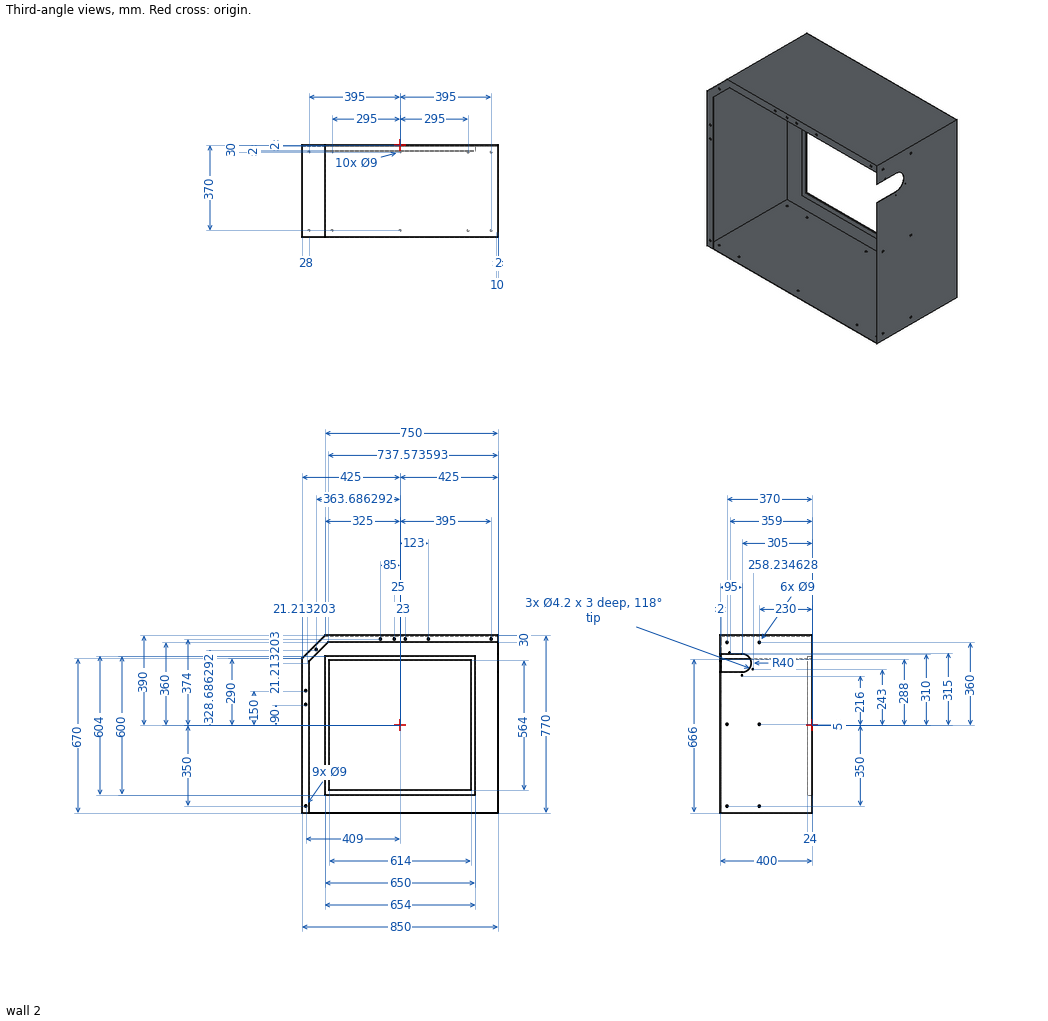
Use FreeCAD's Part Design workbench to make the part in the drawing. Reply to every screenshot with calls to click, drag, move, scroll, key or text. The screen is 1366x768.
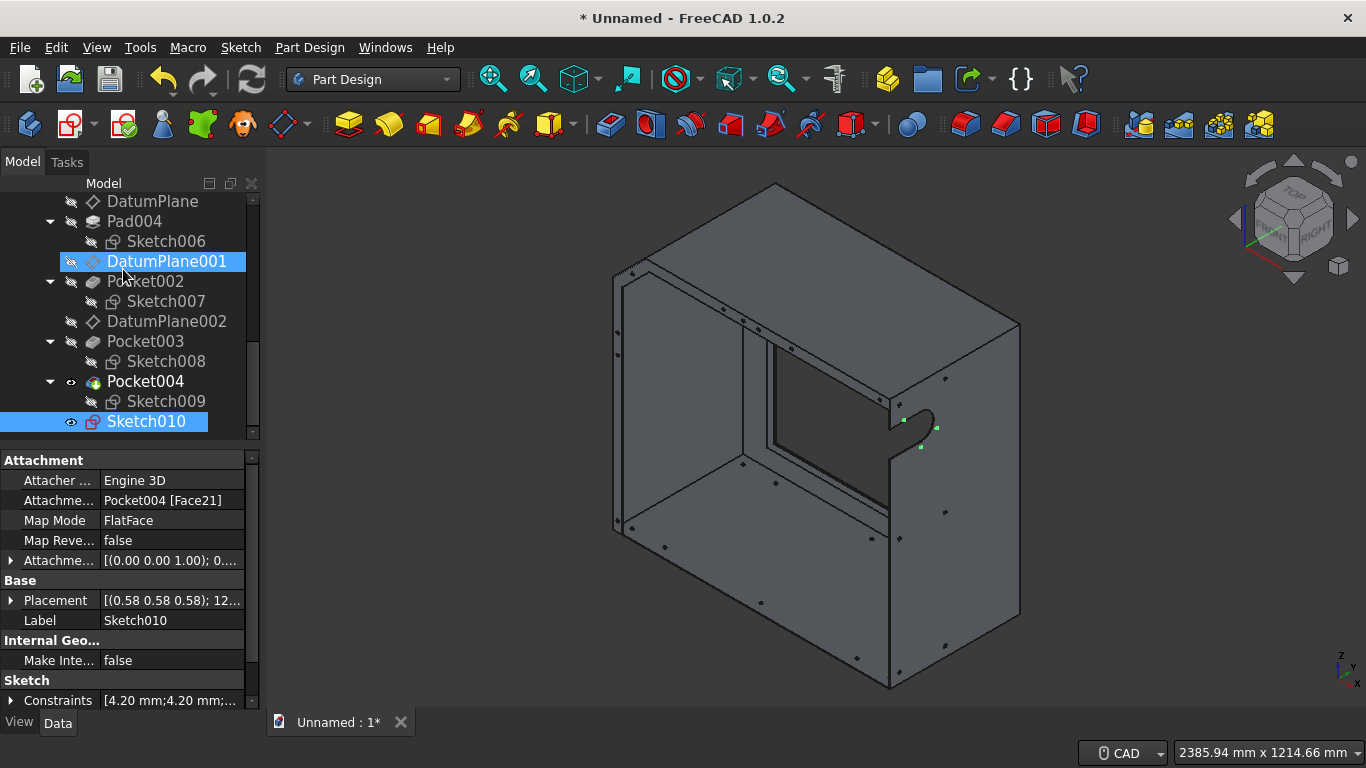
click(652, 124)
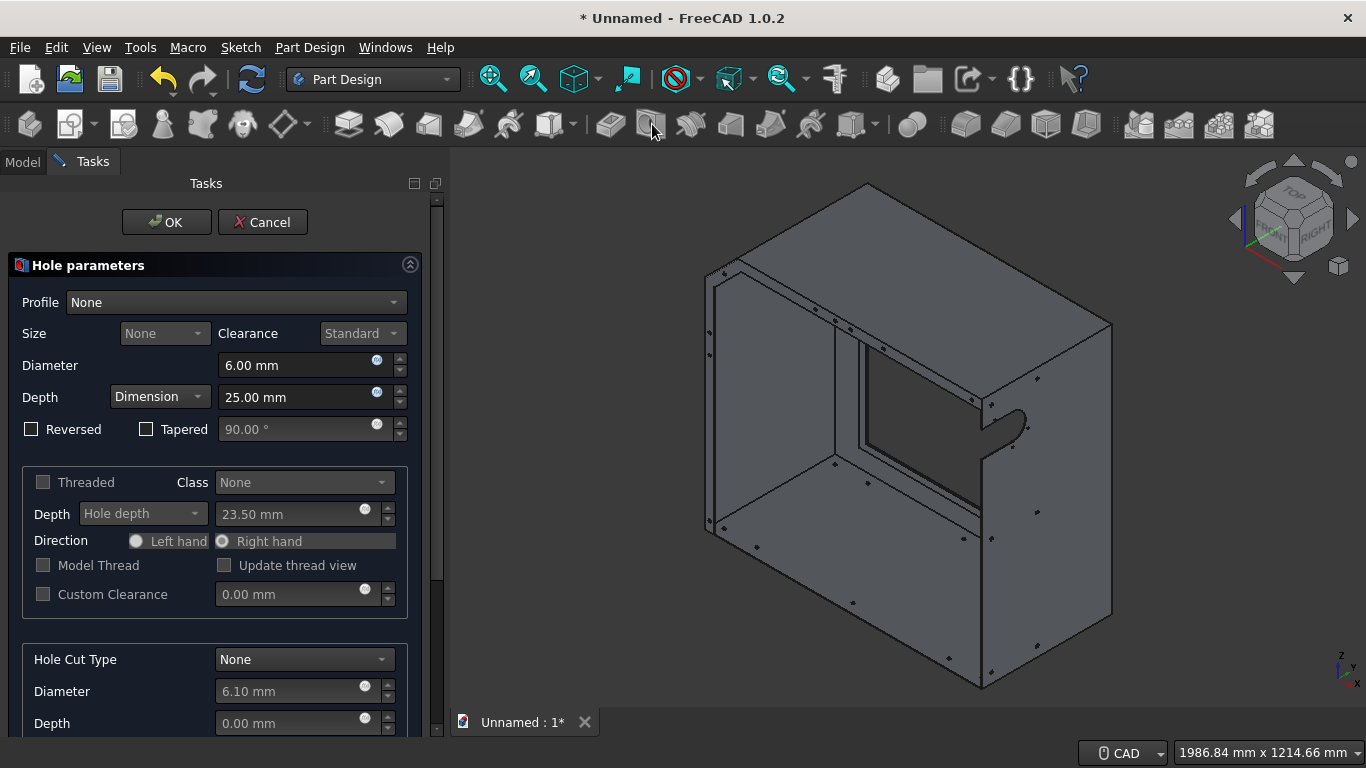
triple_click(305, 365)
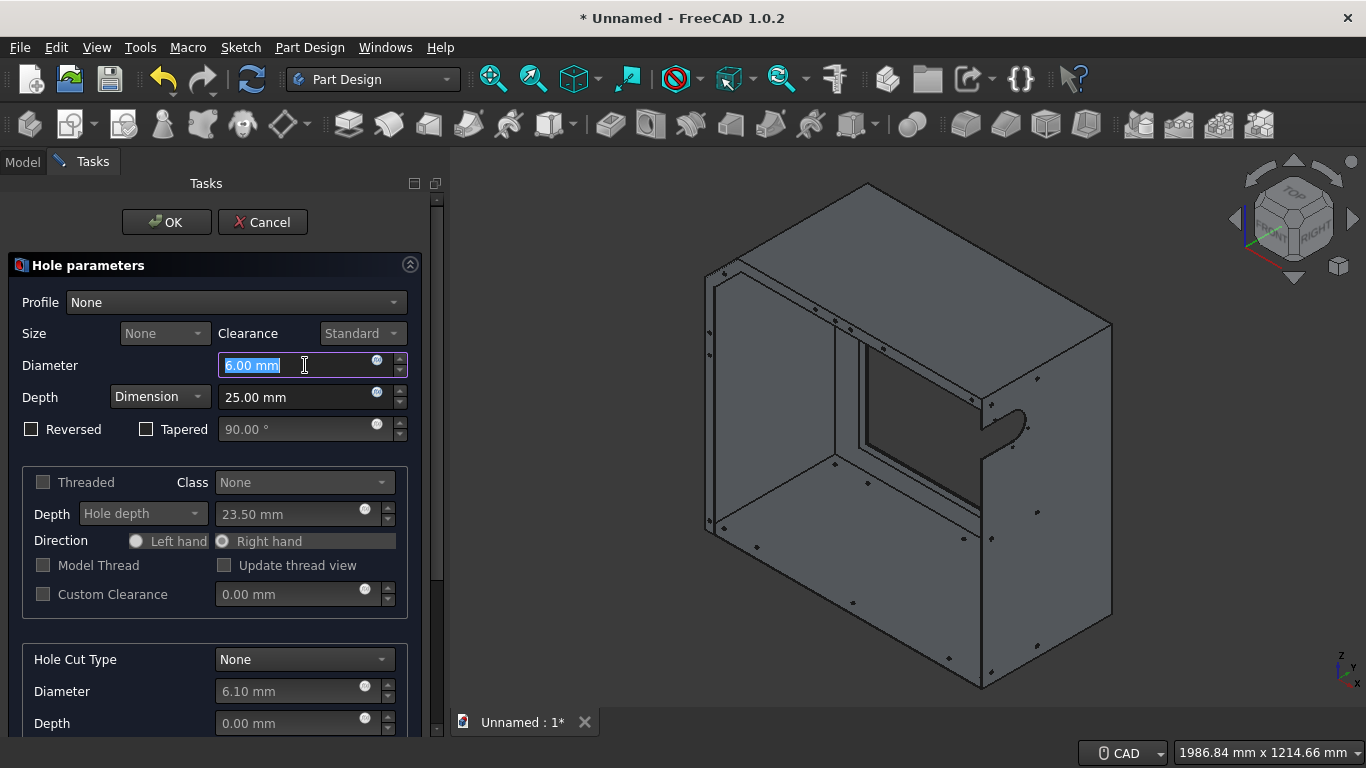
text(4.2)
key(Tab)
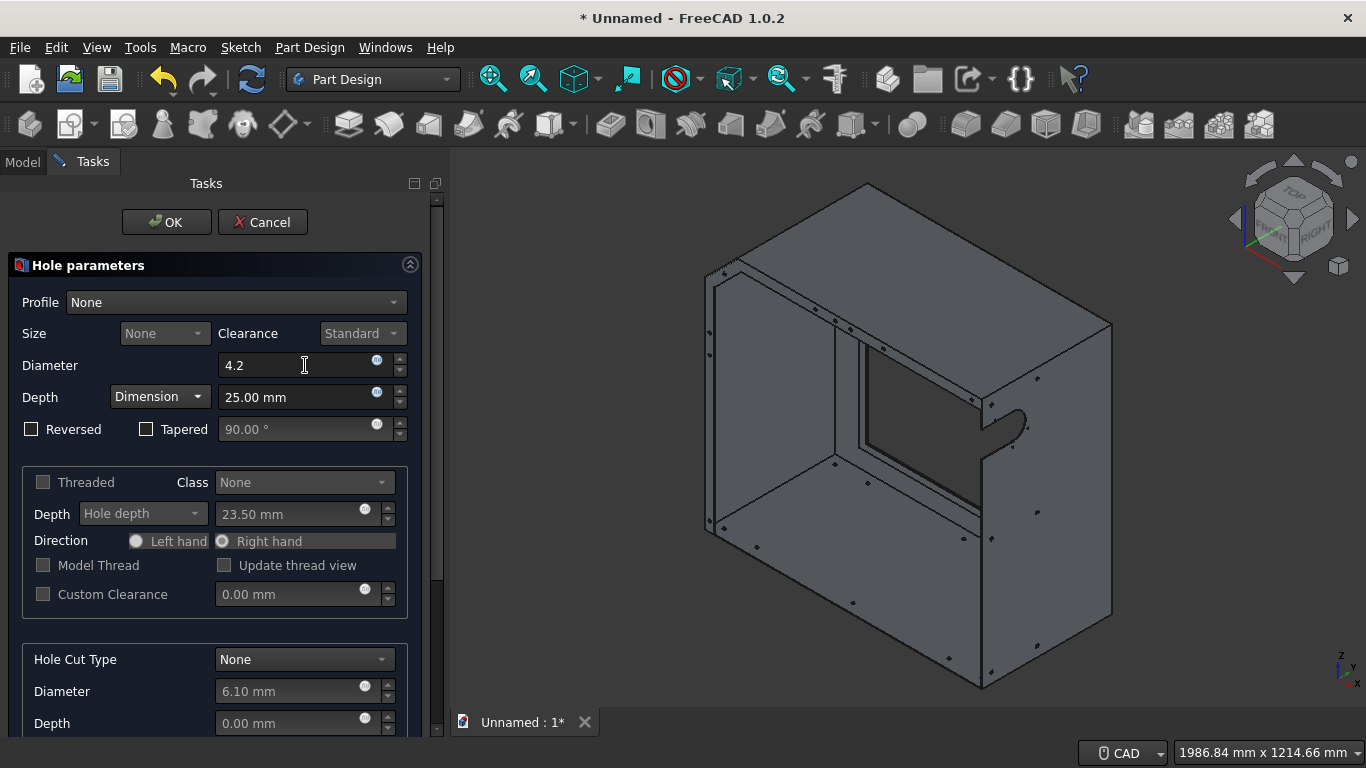
triple_click(305, 397)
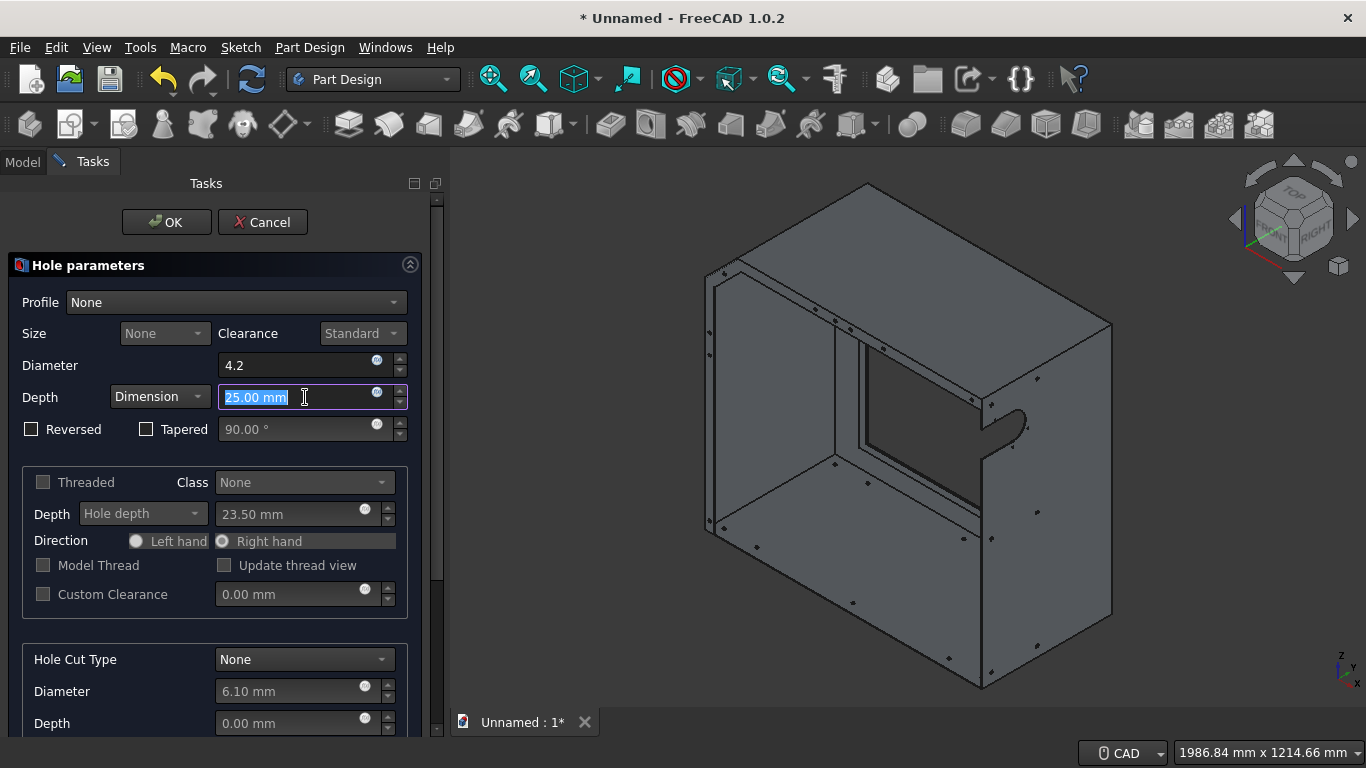
text(3)
key(Tab)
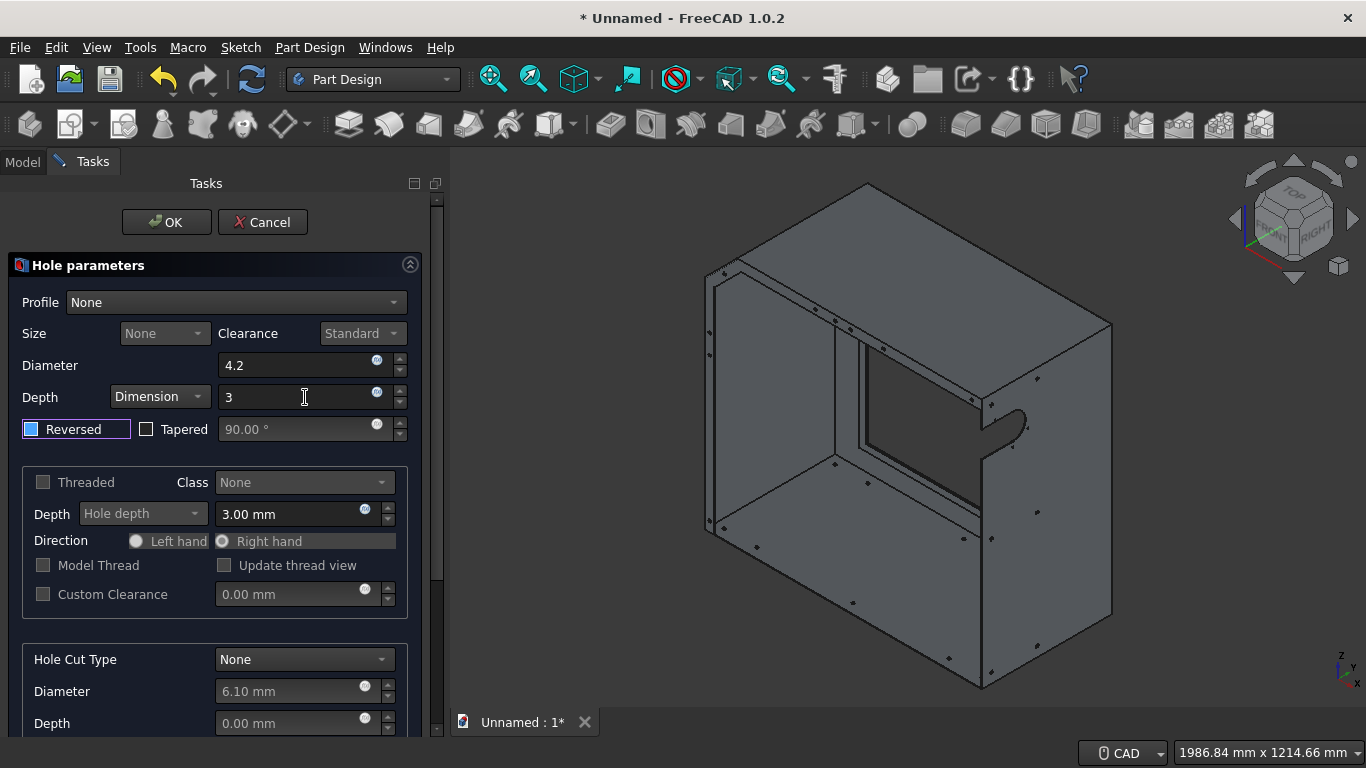
click(167, 222)